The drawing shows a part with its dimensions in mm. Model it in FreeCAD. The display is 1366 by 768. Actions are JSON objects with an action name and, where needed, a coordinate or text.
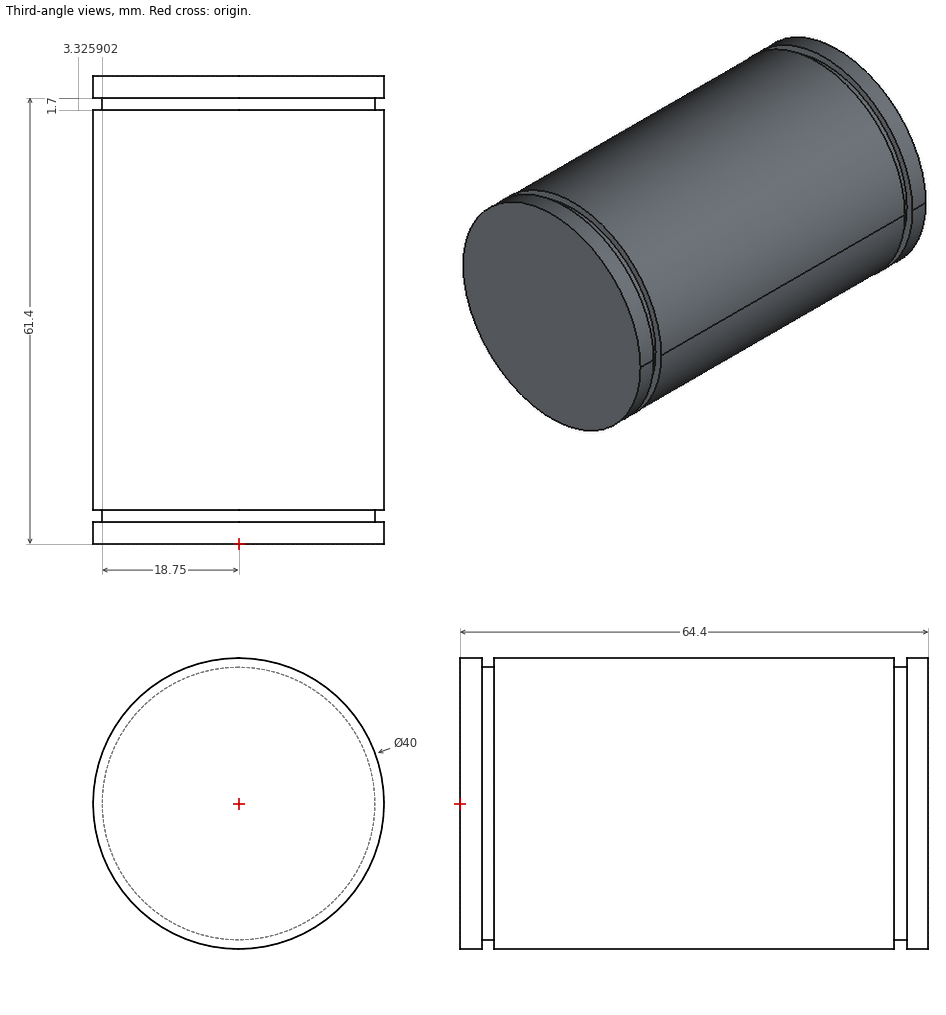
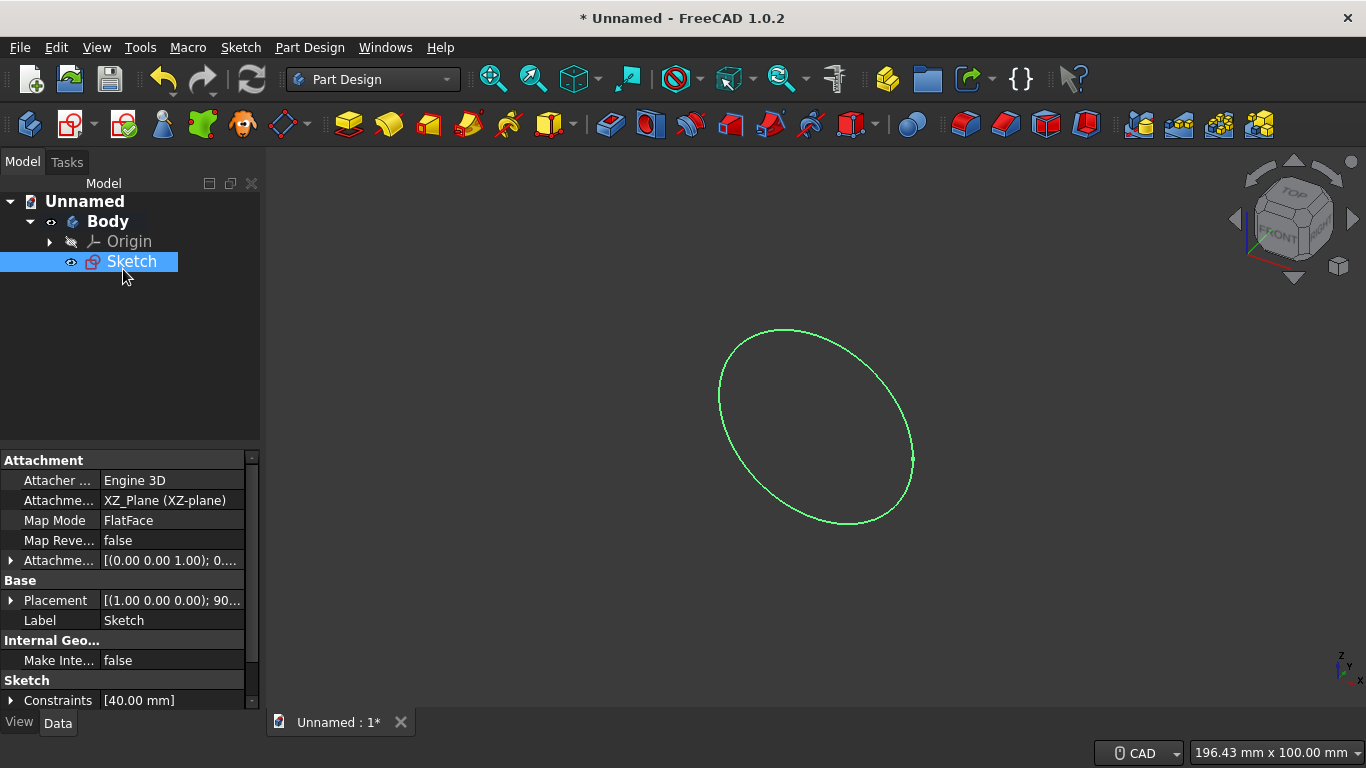
{"action": "left_click", "coordinate": [350, 124]}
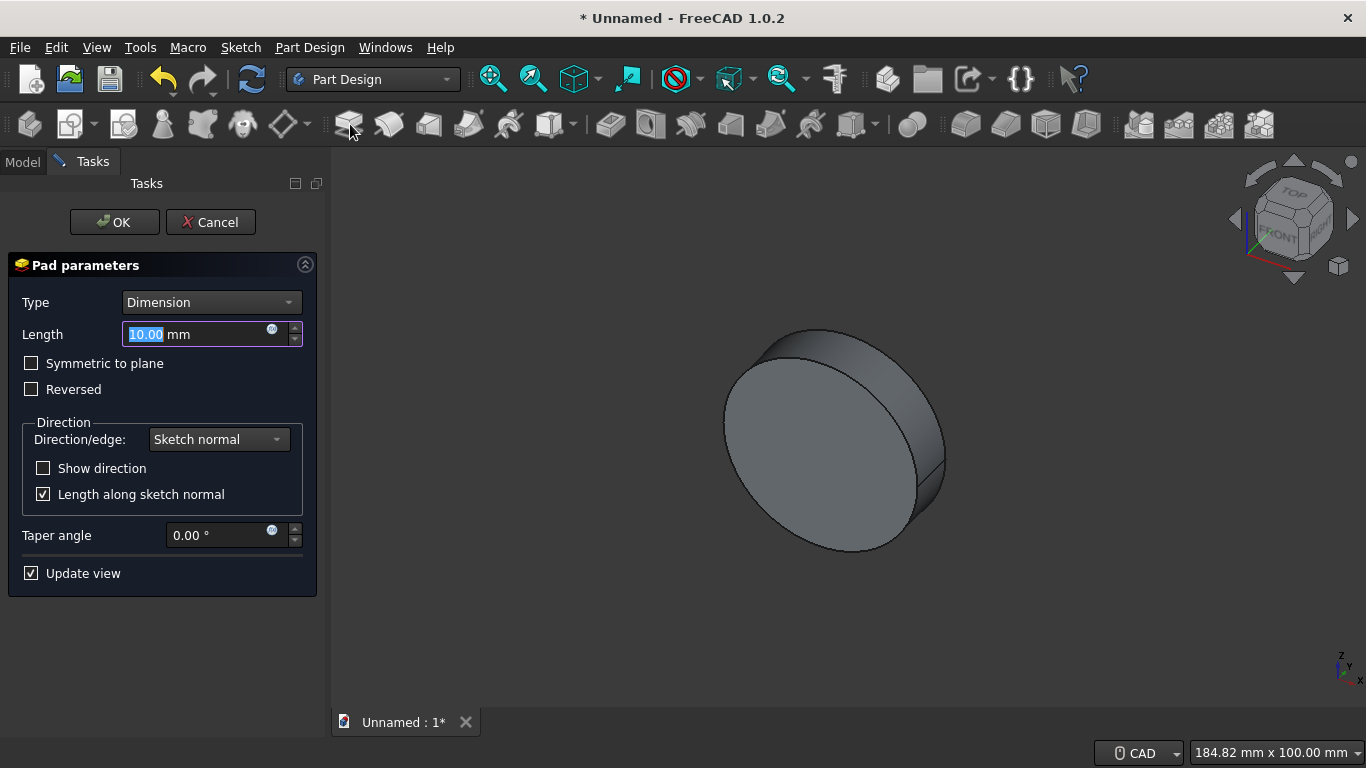
{"action": "type", "text": "64.4"}
{"action": "key", "text": "Tab"}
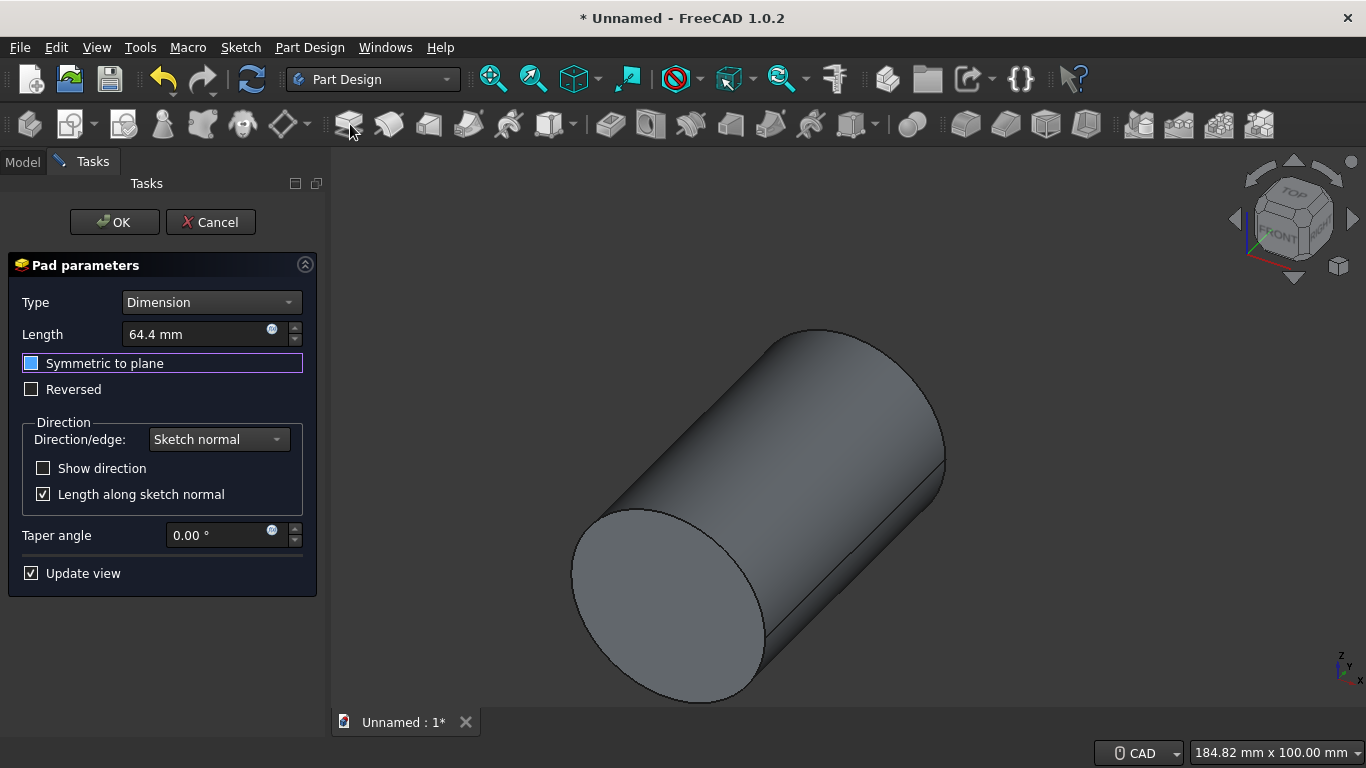
{"action": "left_click", "coordinate": [30, 389]}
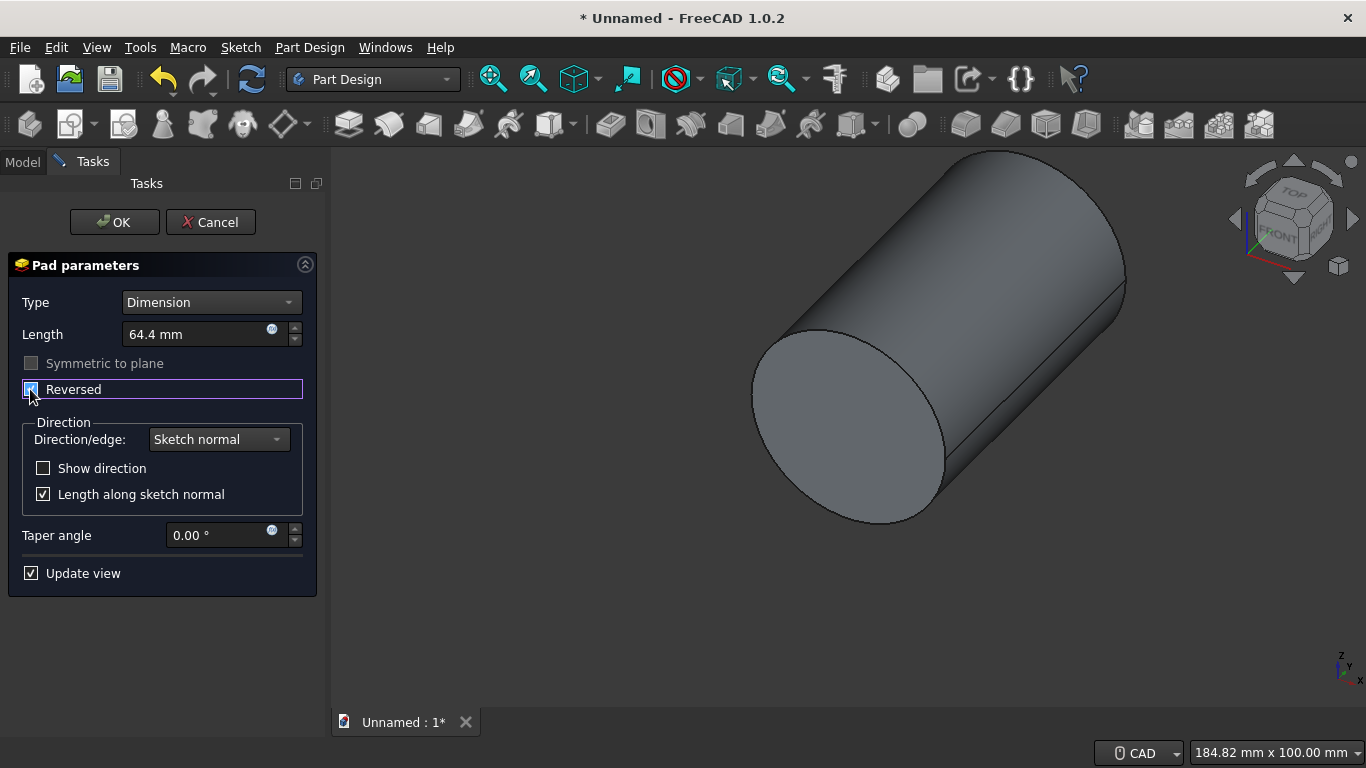
{"action": "left_click", "coordinate": [115, 222]}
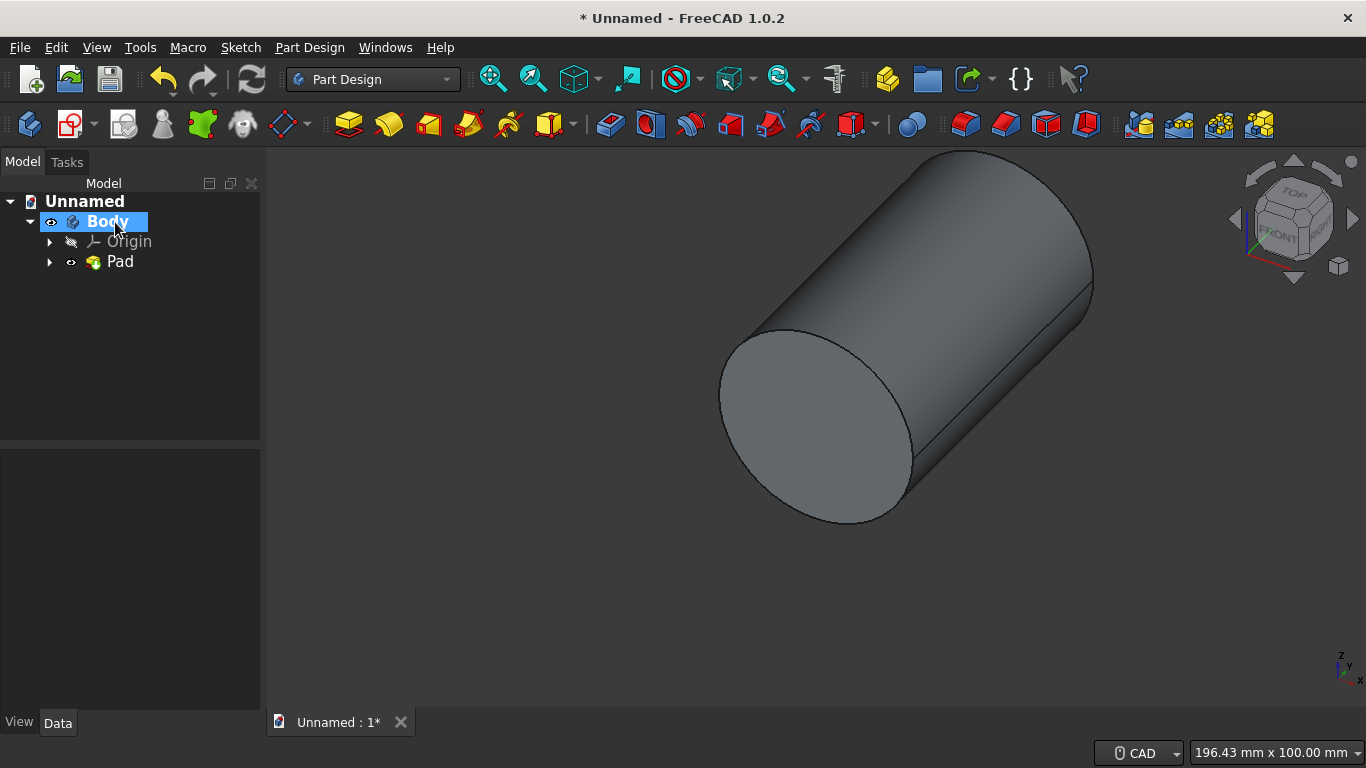
{"action": "left_click", "coordinate": [494, 80]}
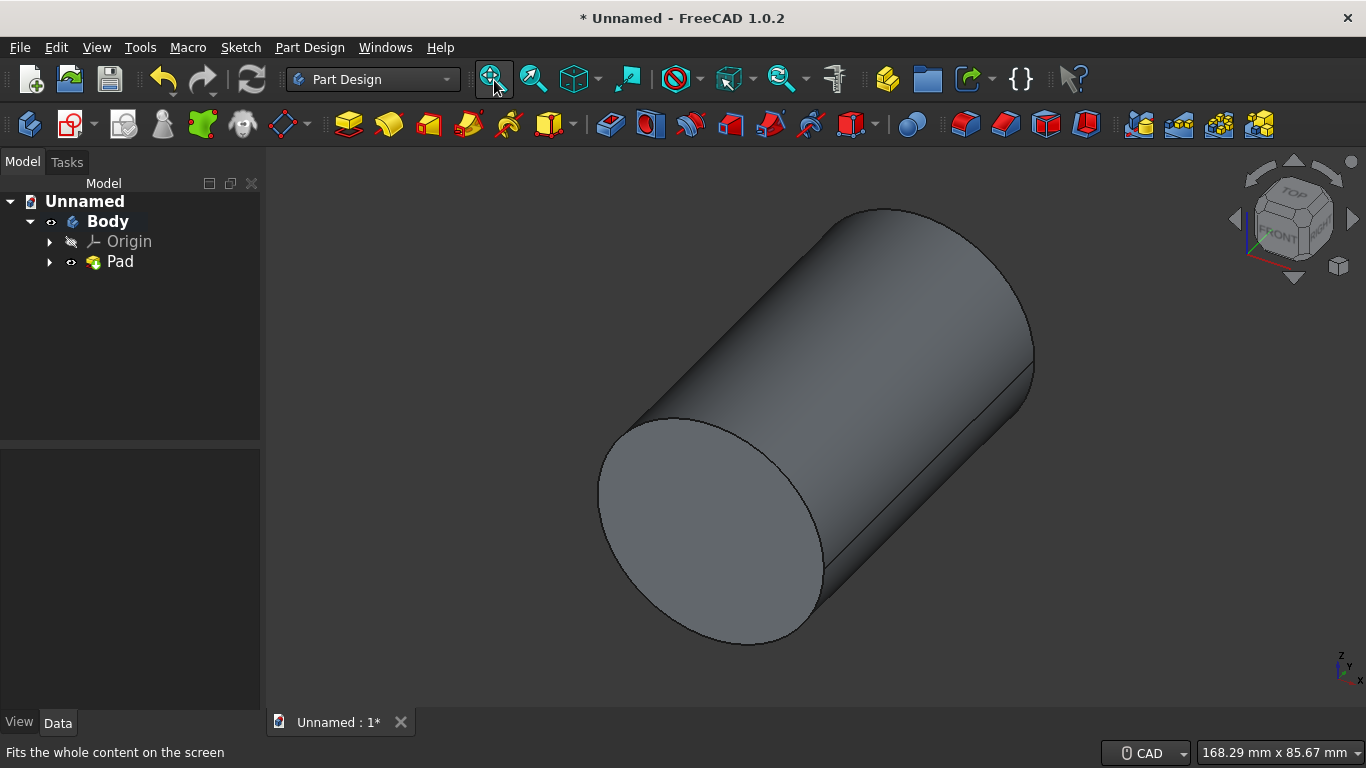
{"action": "left_click", "coordinate": [70, 124]}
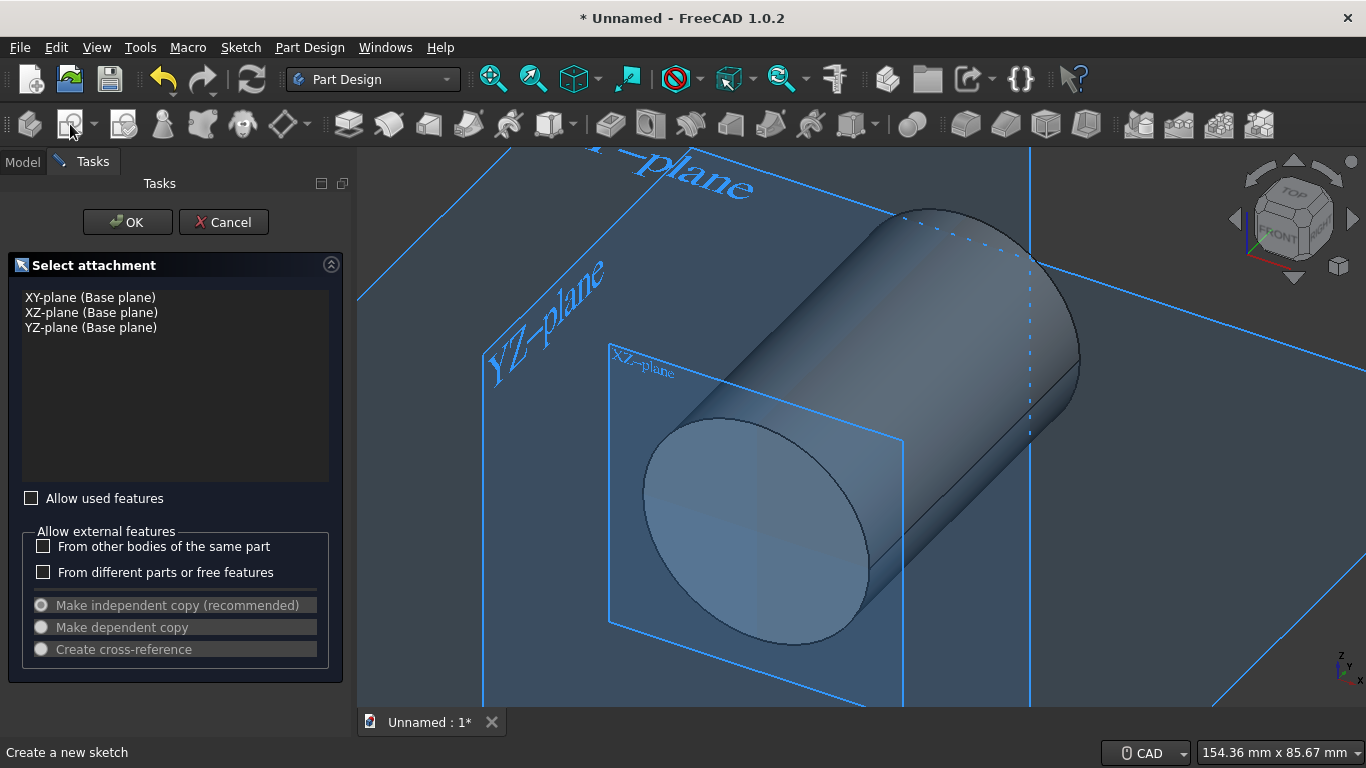
{"action": "left_click", "coordinate": [82, 298]}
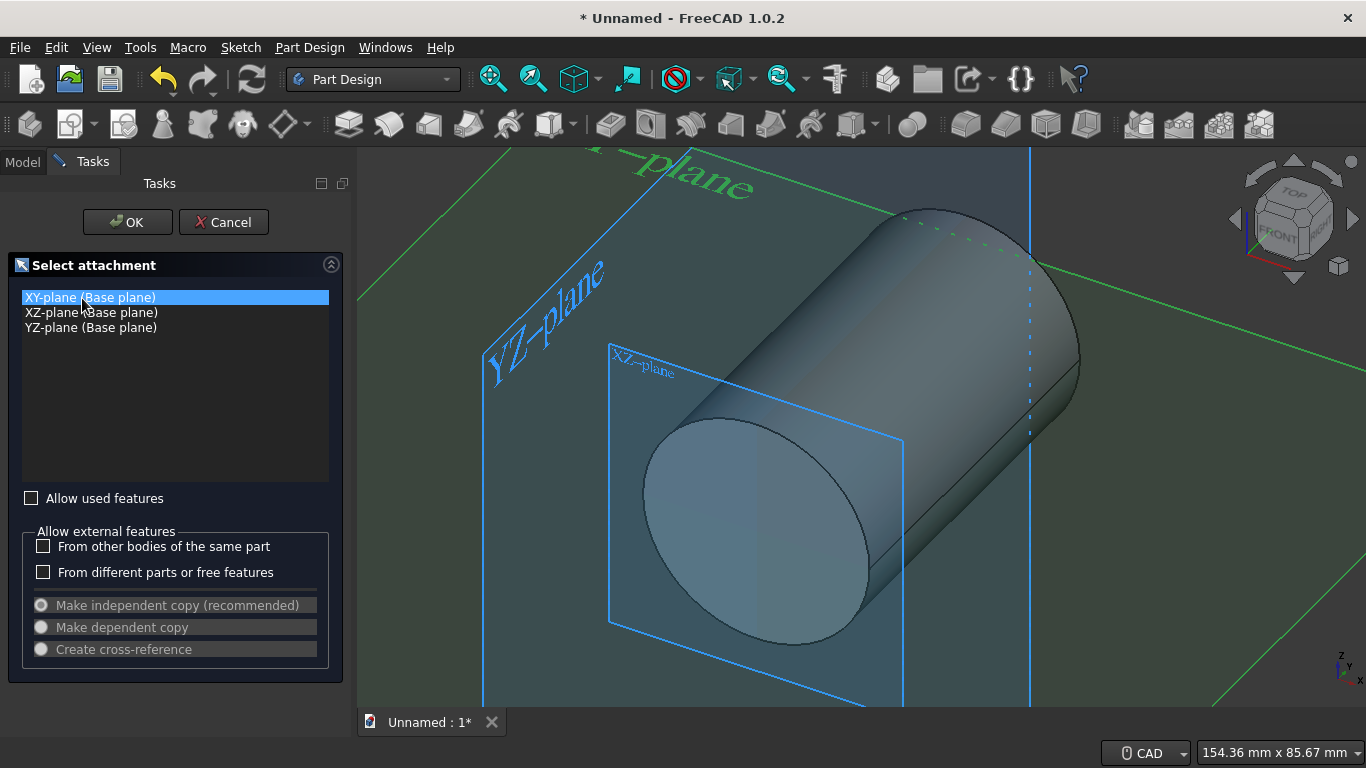
{"action": "left_click", "coordinate": [128, 222]}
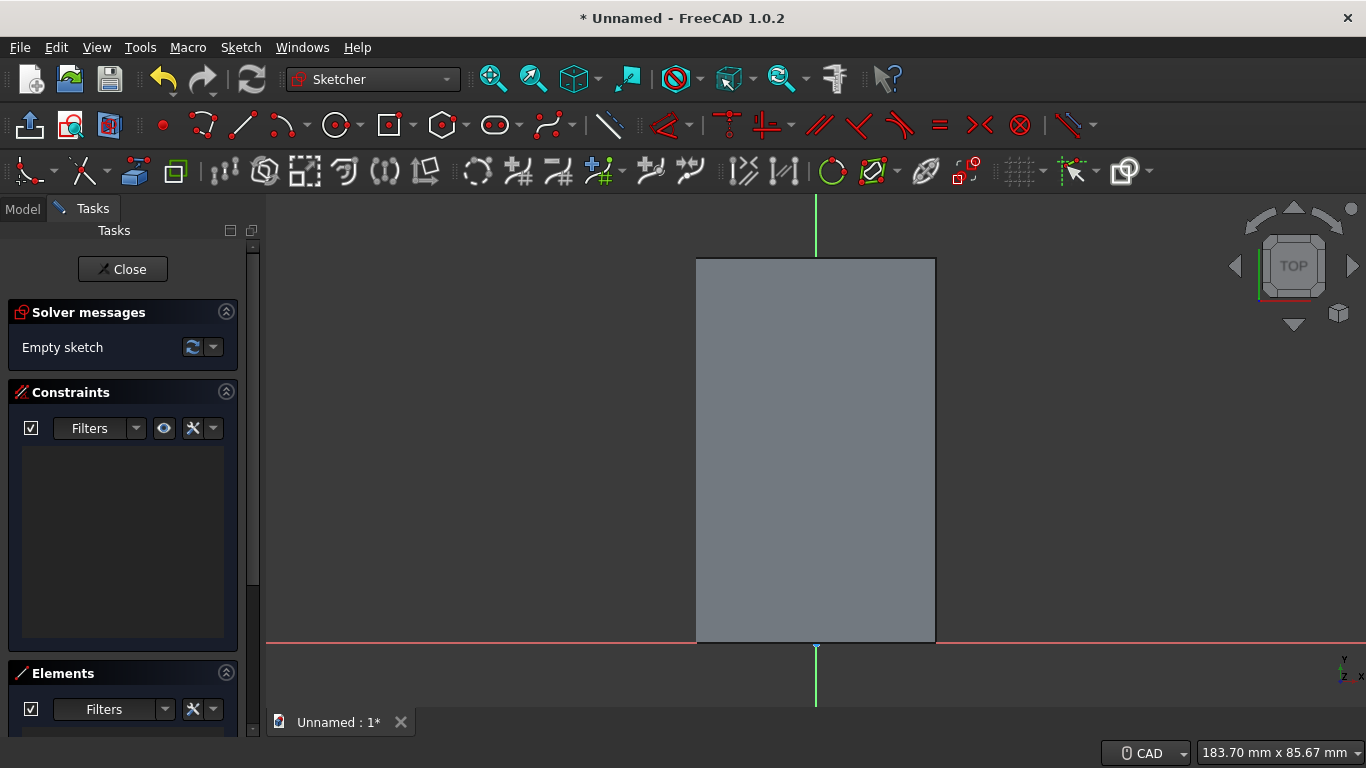
{"action": "left_click", "coordinate": [110, 126]}